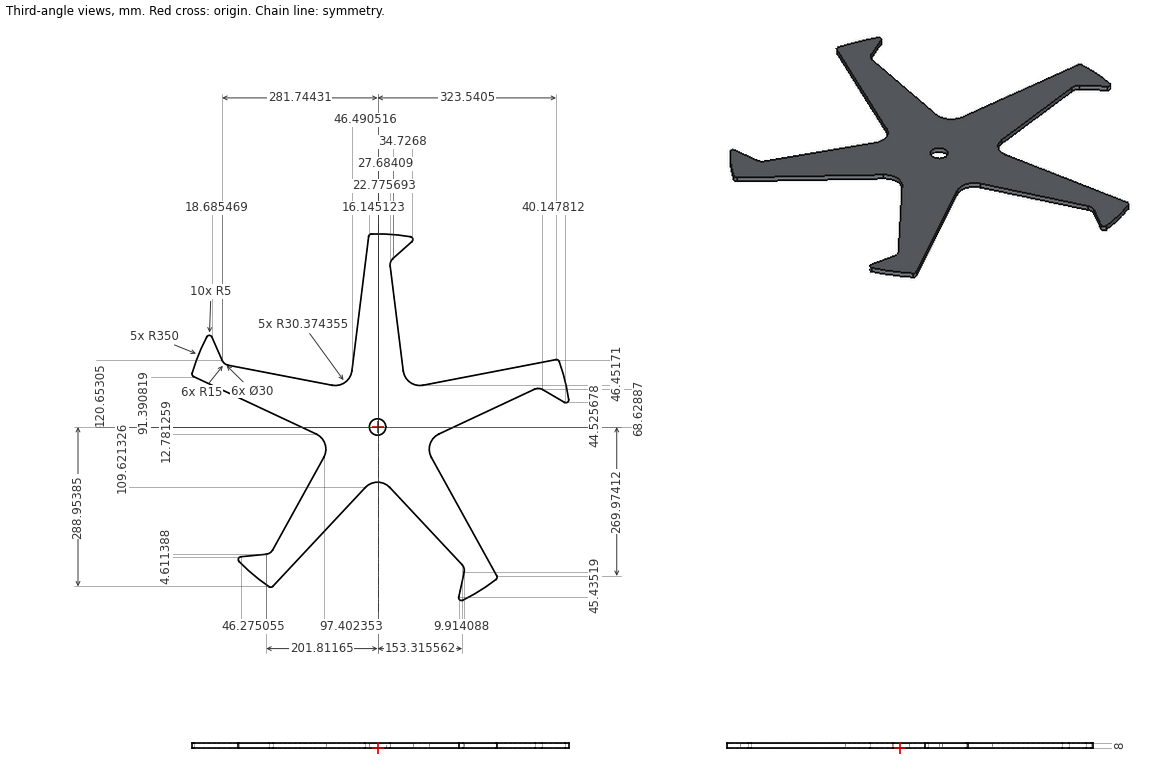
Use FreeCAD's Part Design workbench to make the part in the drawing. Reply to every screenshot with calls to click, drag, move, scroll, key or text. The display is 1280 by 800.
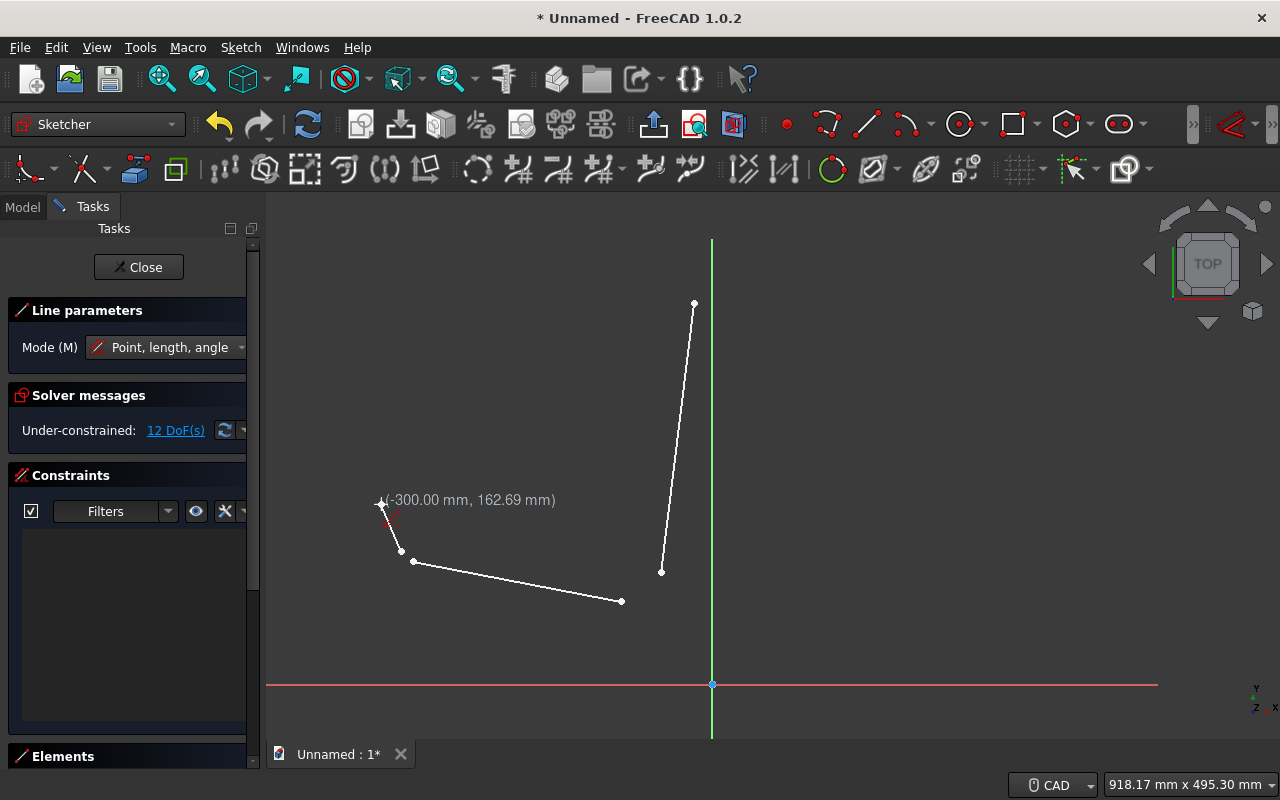
click(344, 584)
click(590, 699)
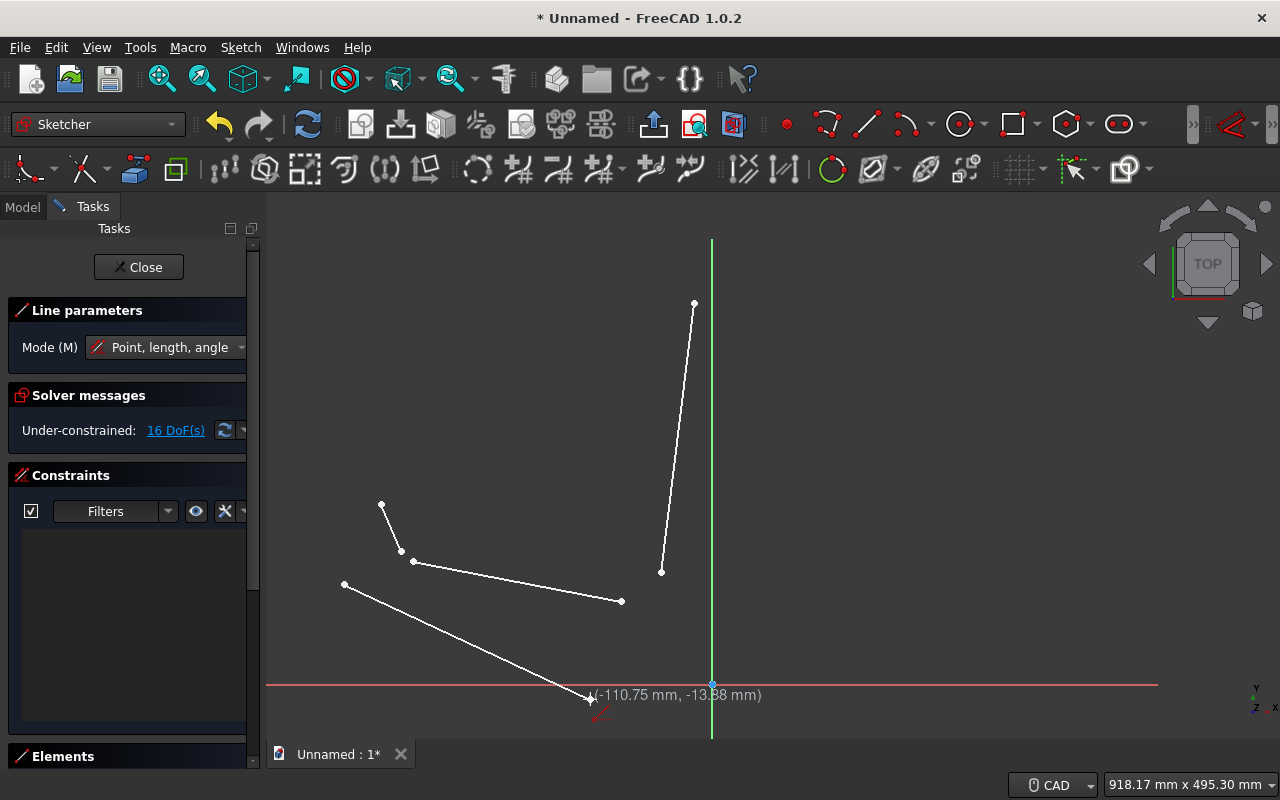
scroll(693, 303, down, 4)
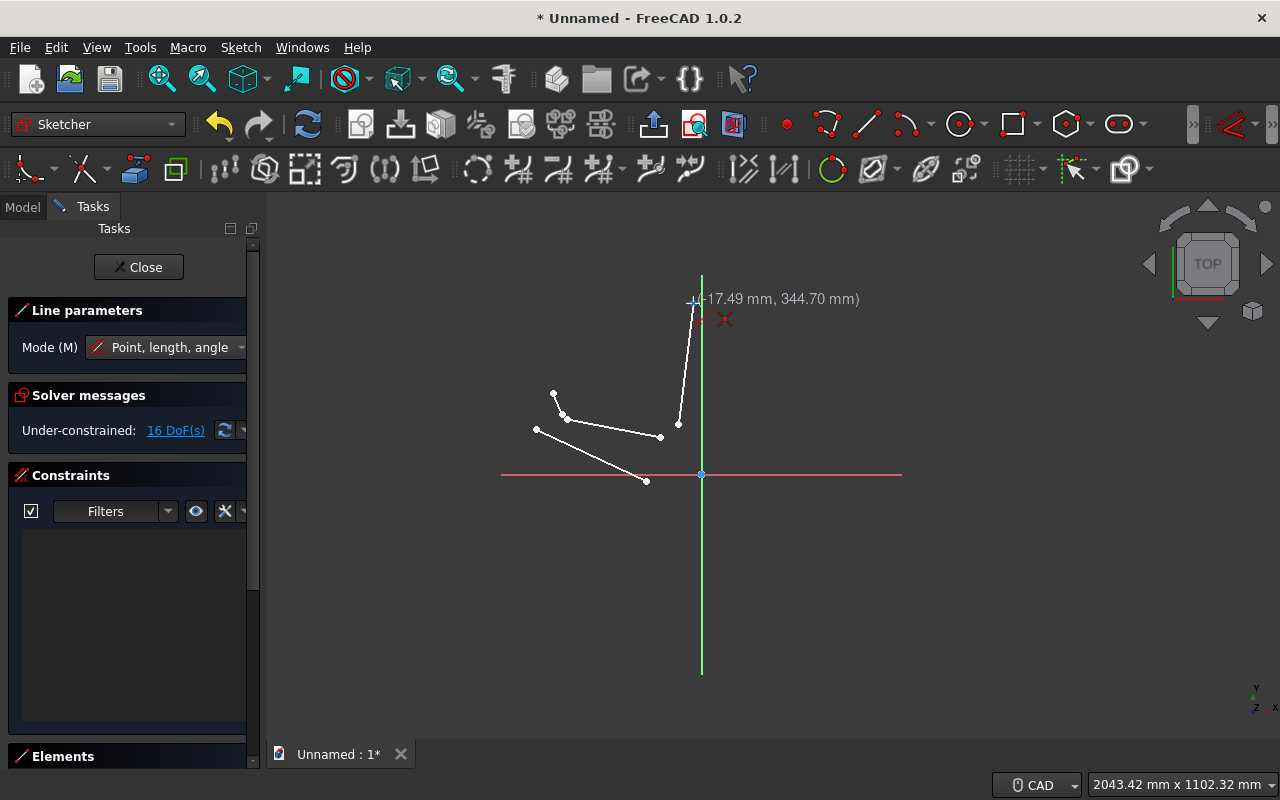
click(654, 502)
click(608, 585)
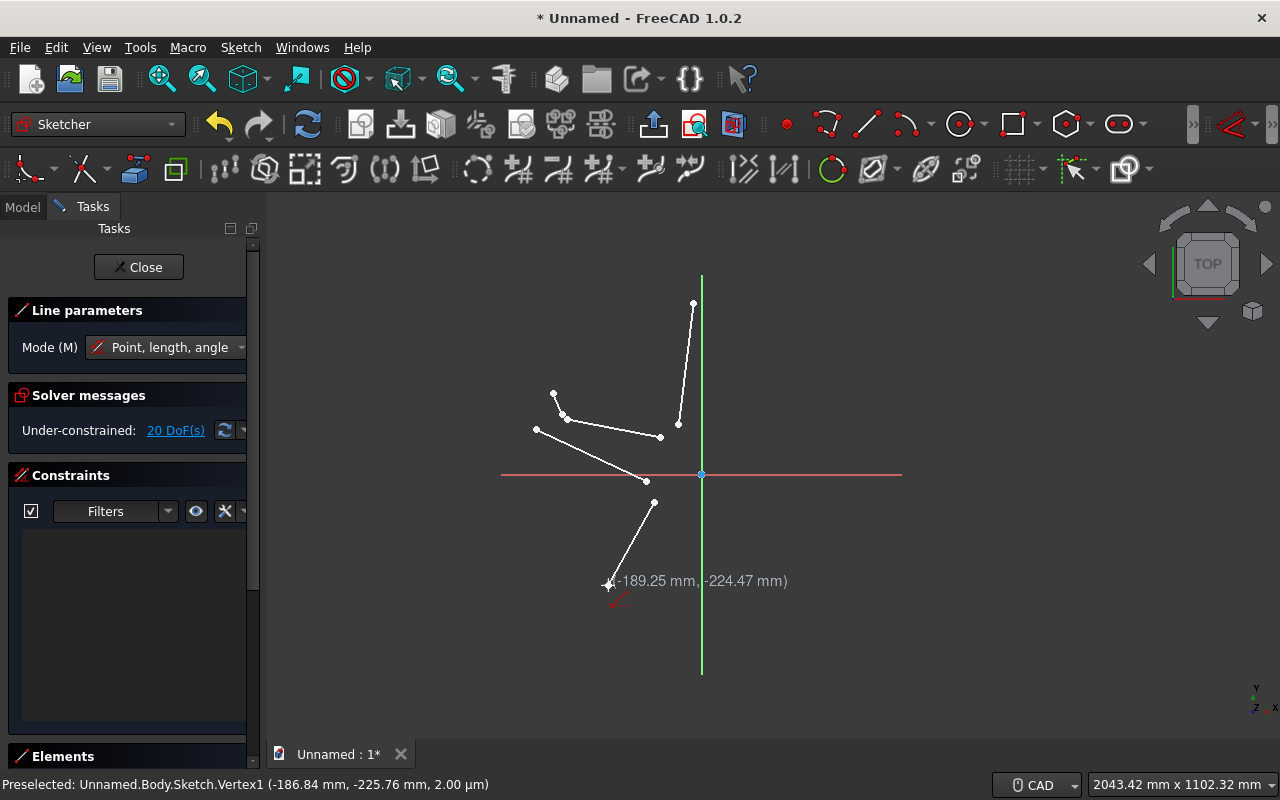
scroll(602, 589, up, 5)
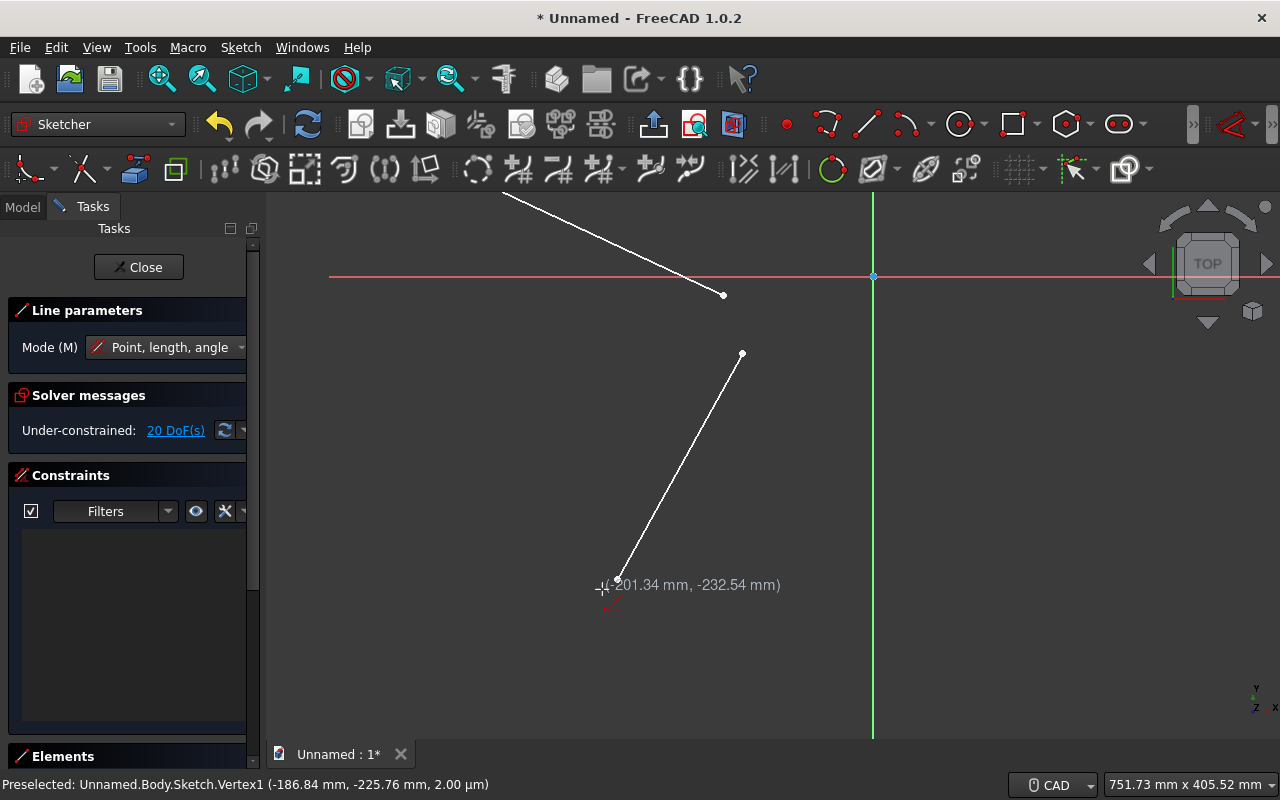
click(601, 588)
click(538, 594)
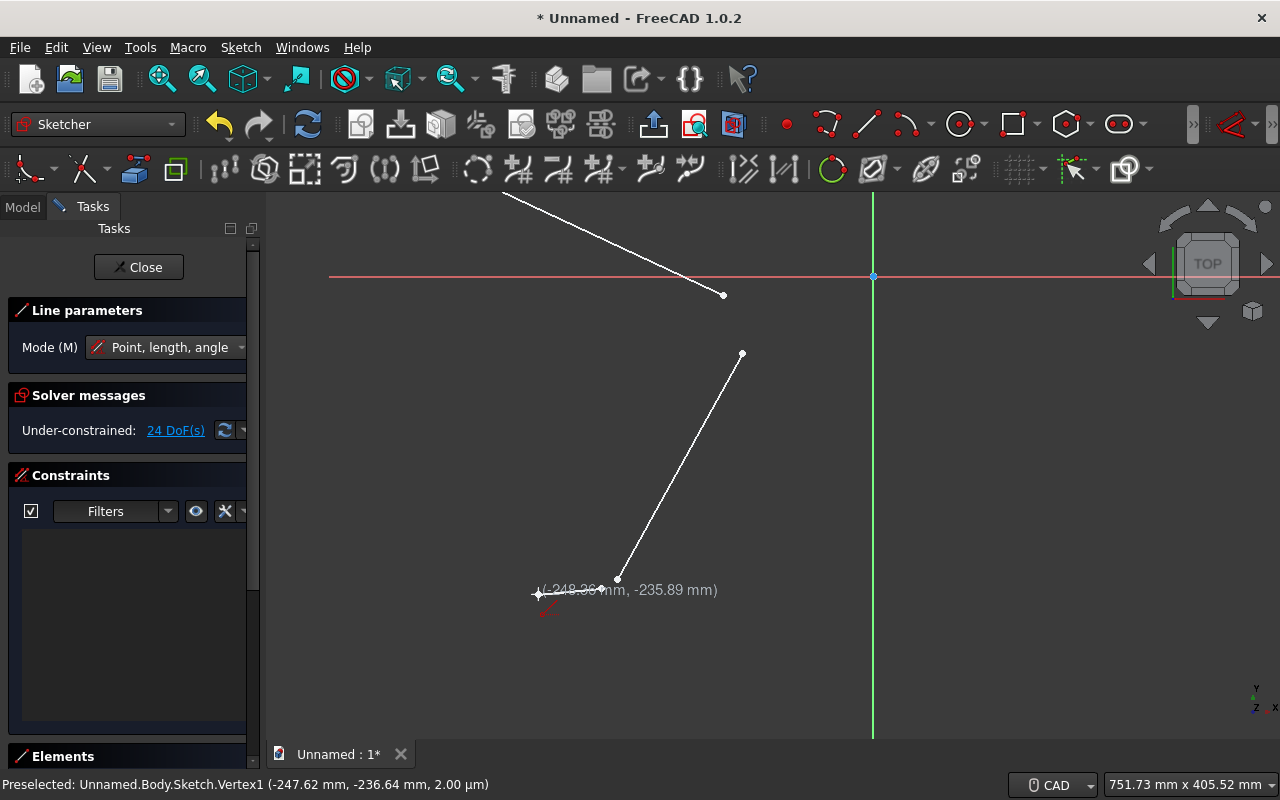
click(617, 667)
click(843, 425)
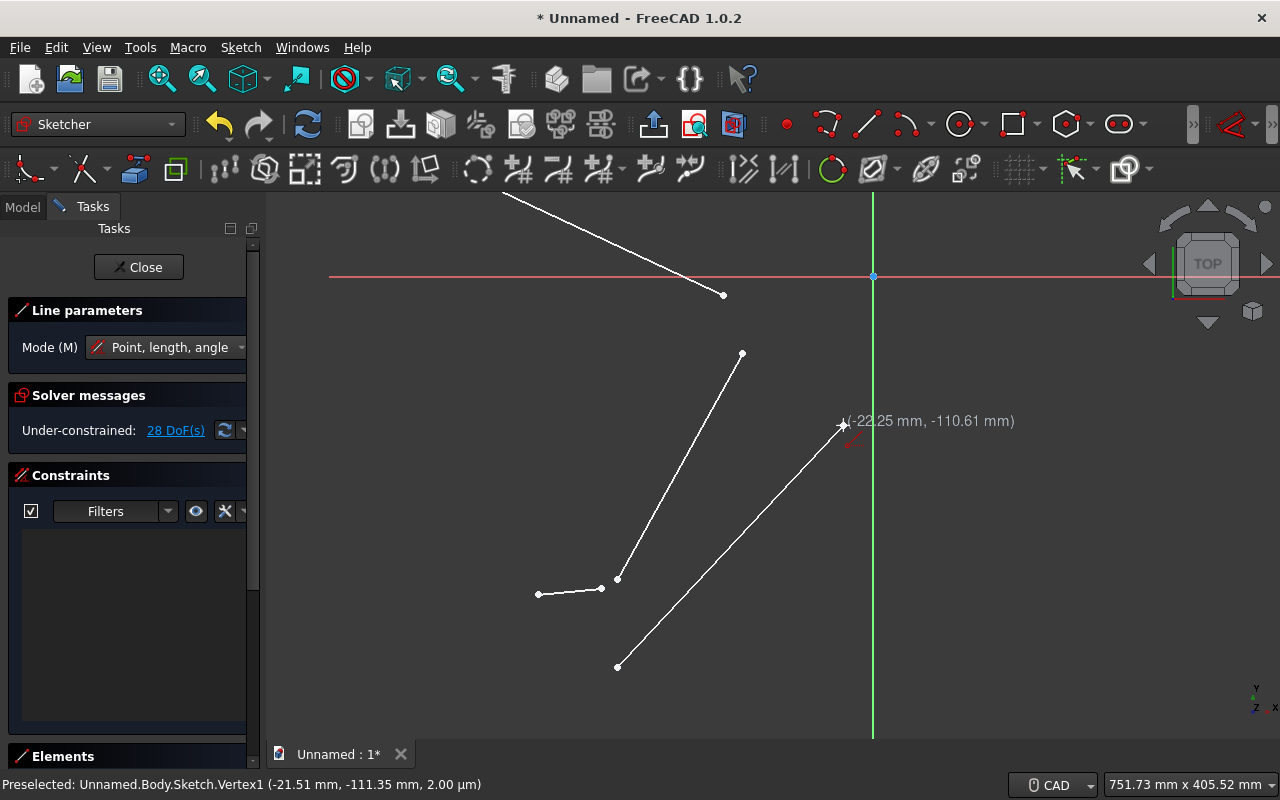
click(903, 425)
click(1080, 614)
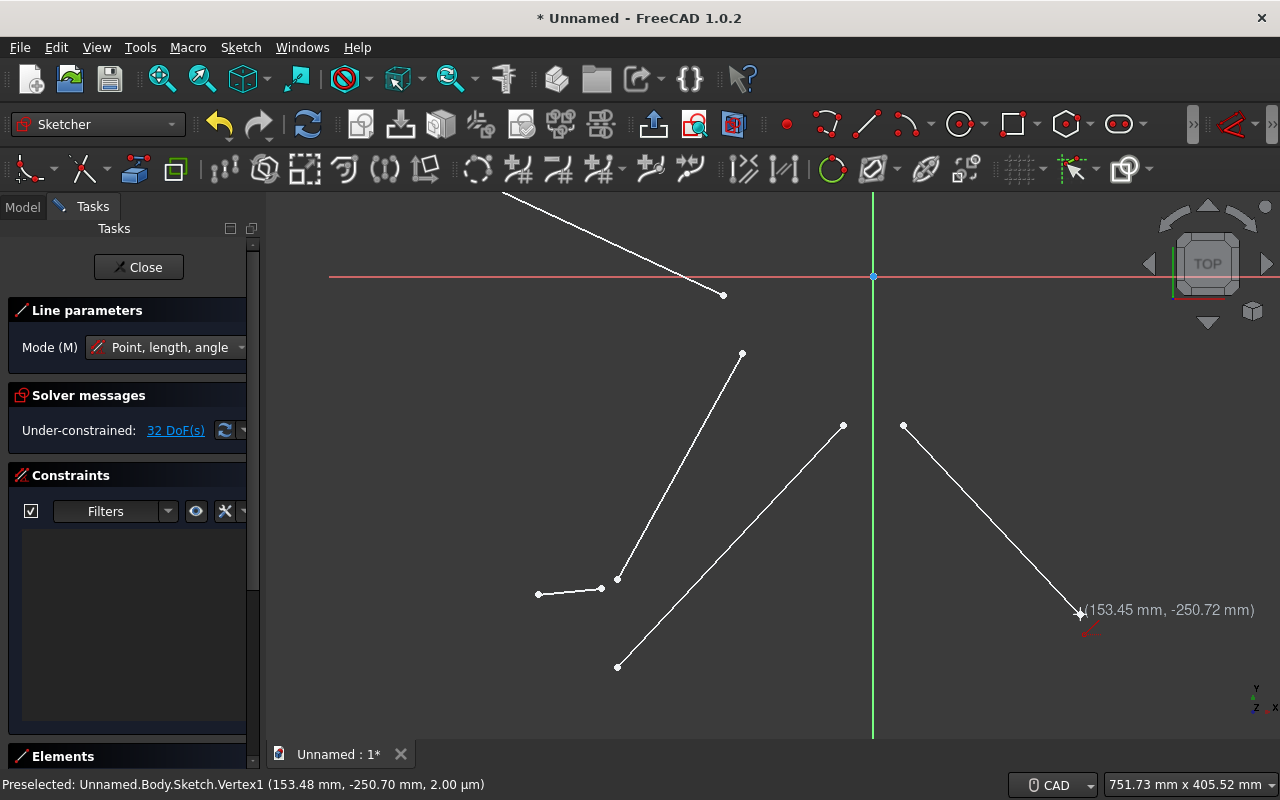
click(1085, 632)
click(1071, 693)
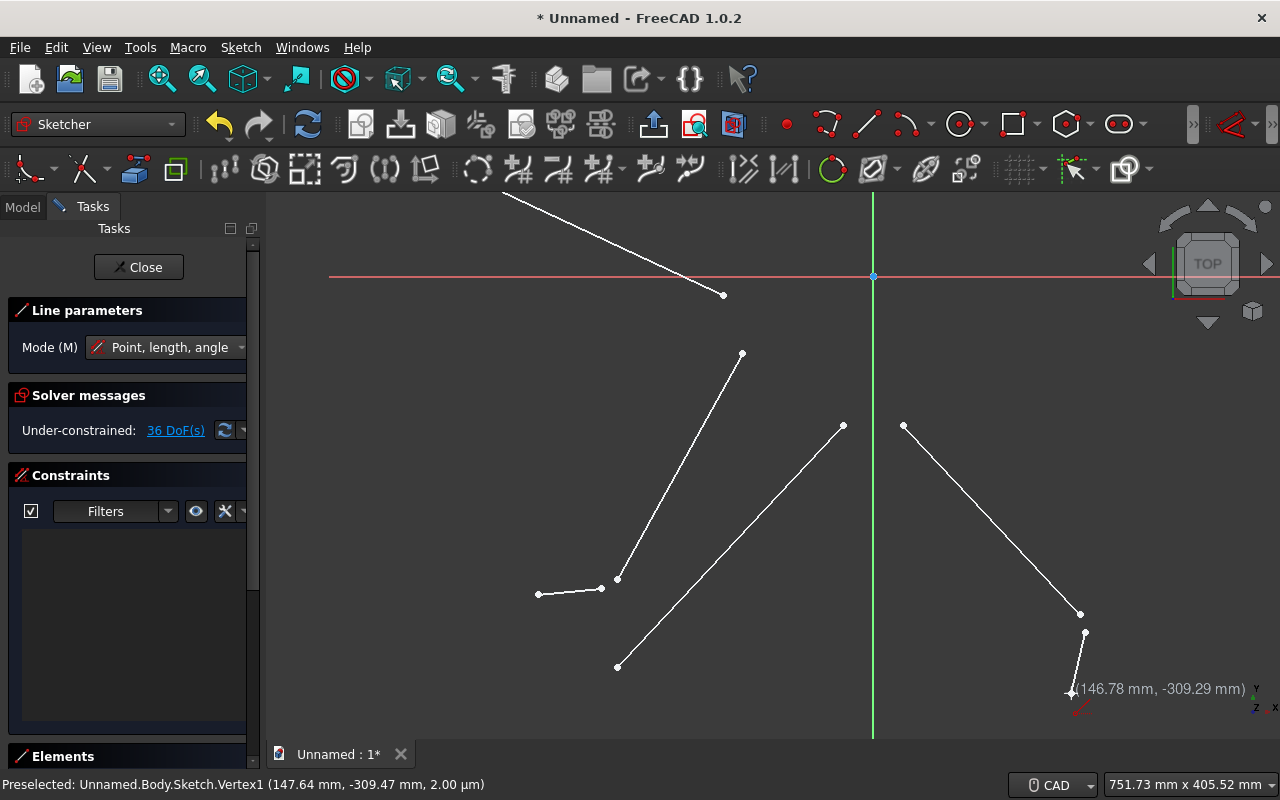
scroll(602, 589, down, 5)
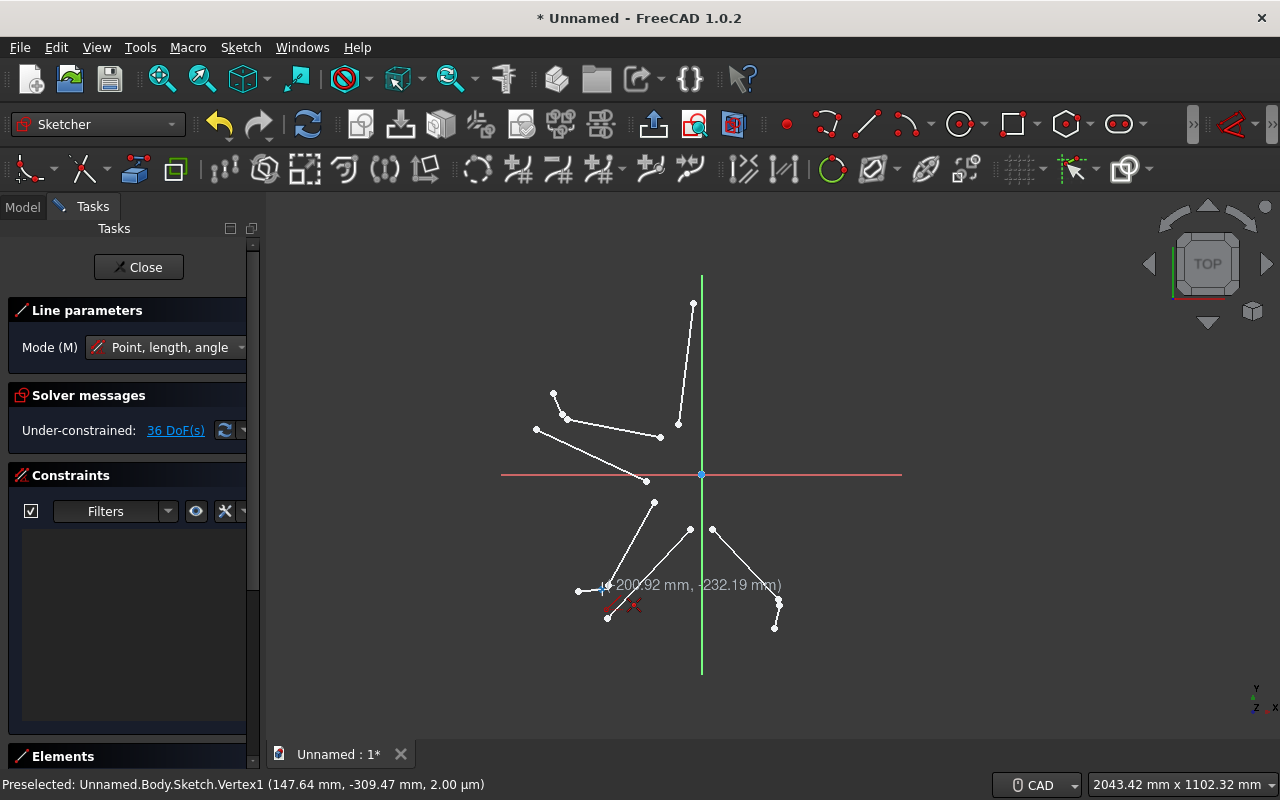
click(809, 609)
click(750, 502)